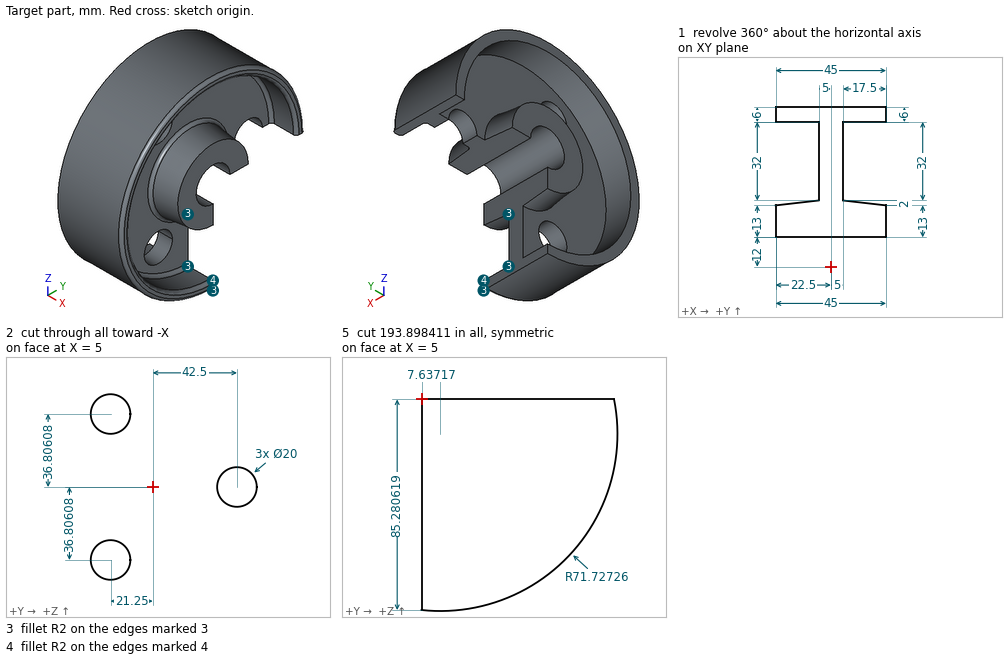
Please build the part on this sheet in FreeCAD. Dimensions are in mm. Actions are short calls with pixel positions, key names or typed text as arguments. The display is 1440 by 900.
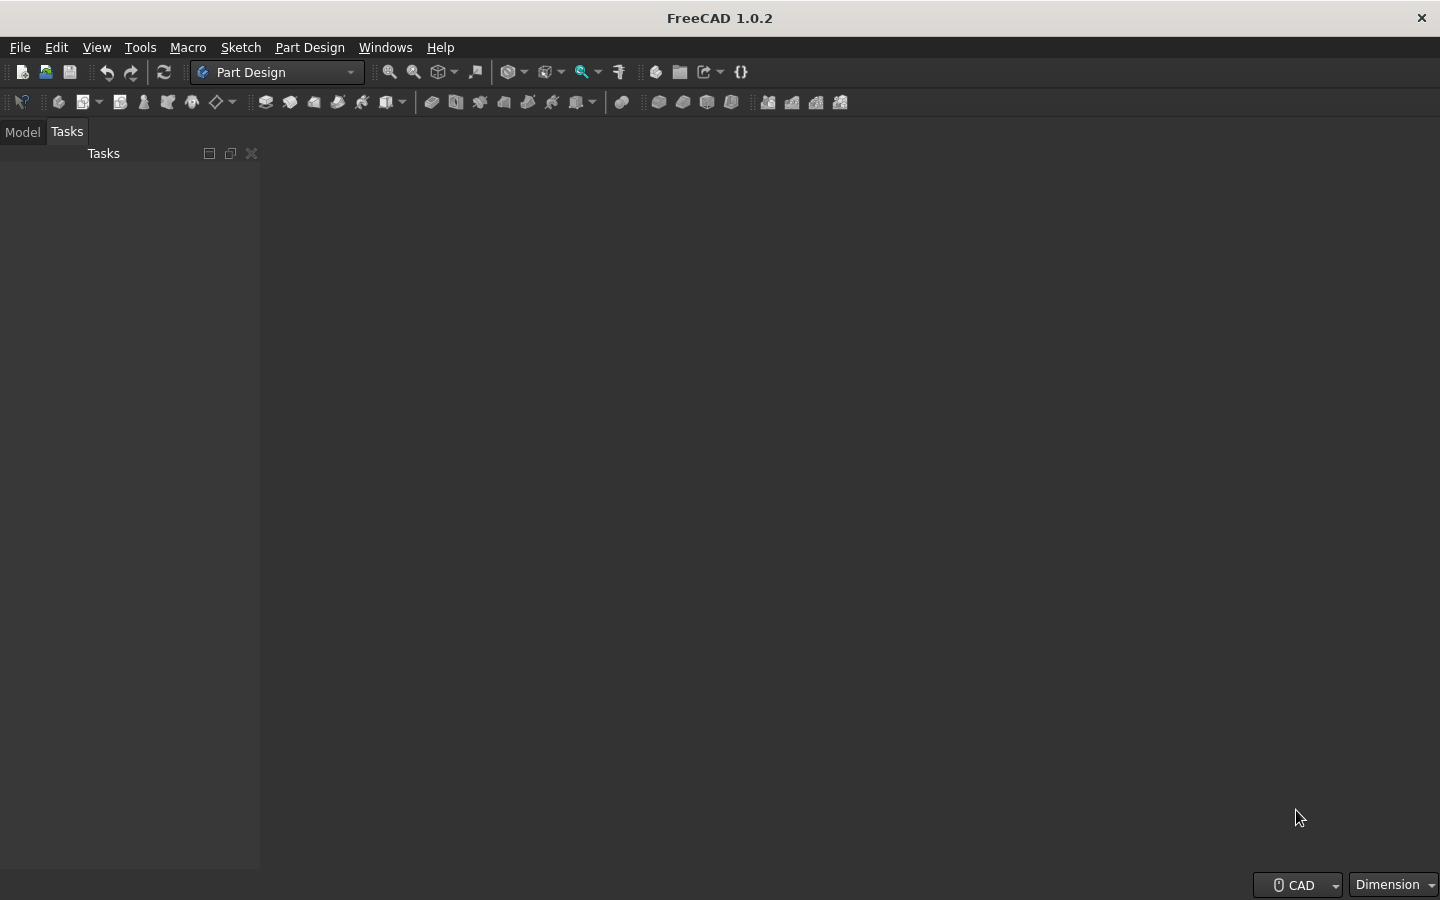
click(22, 72)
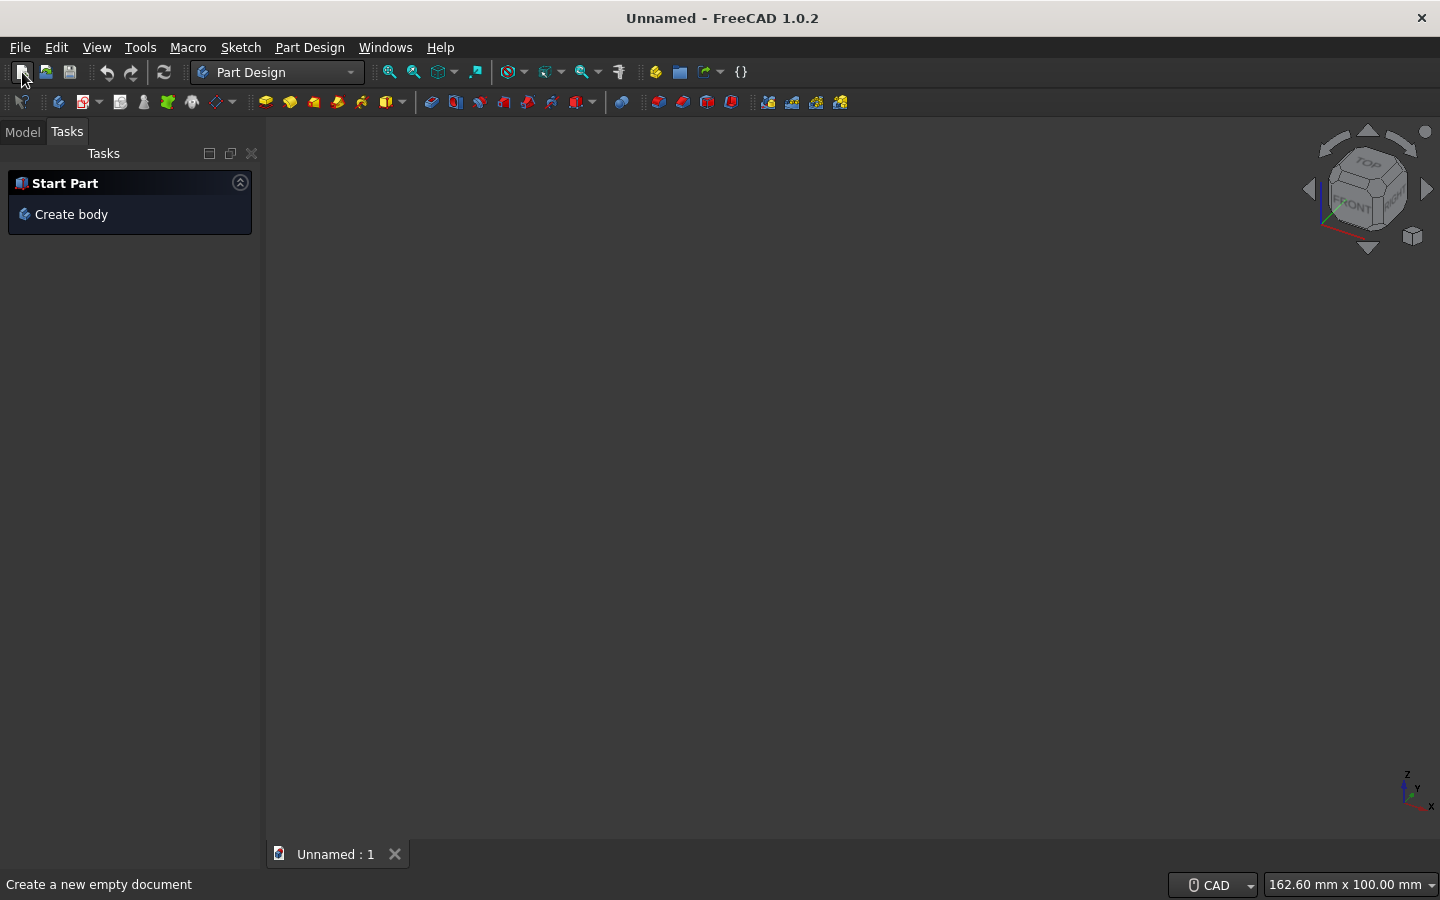
click(84, 102)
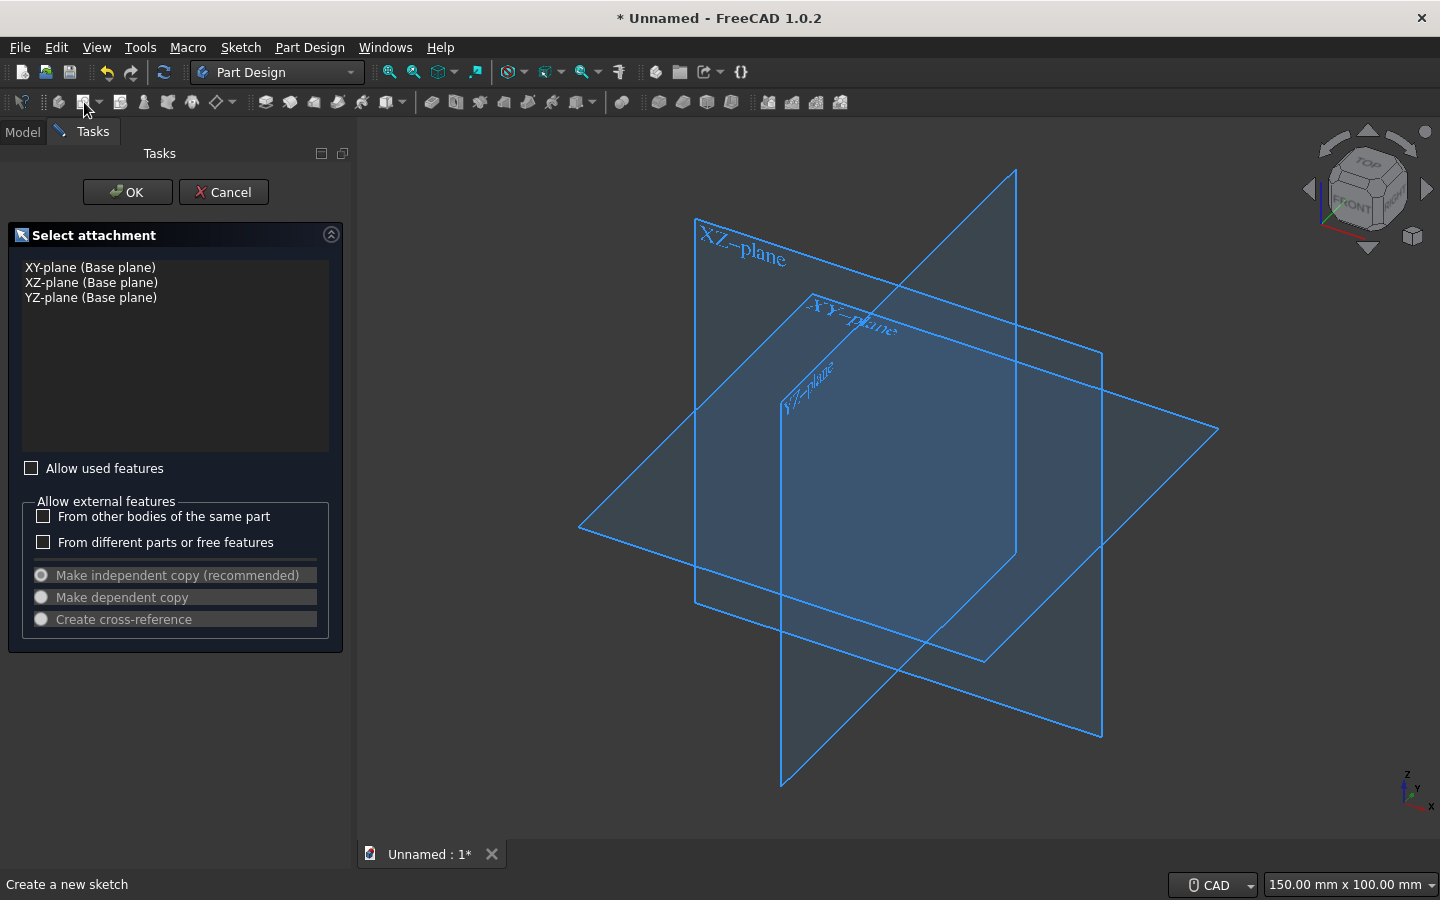
click(82, 268)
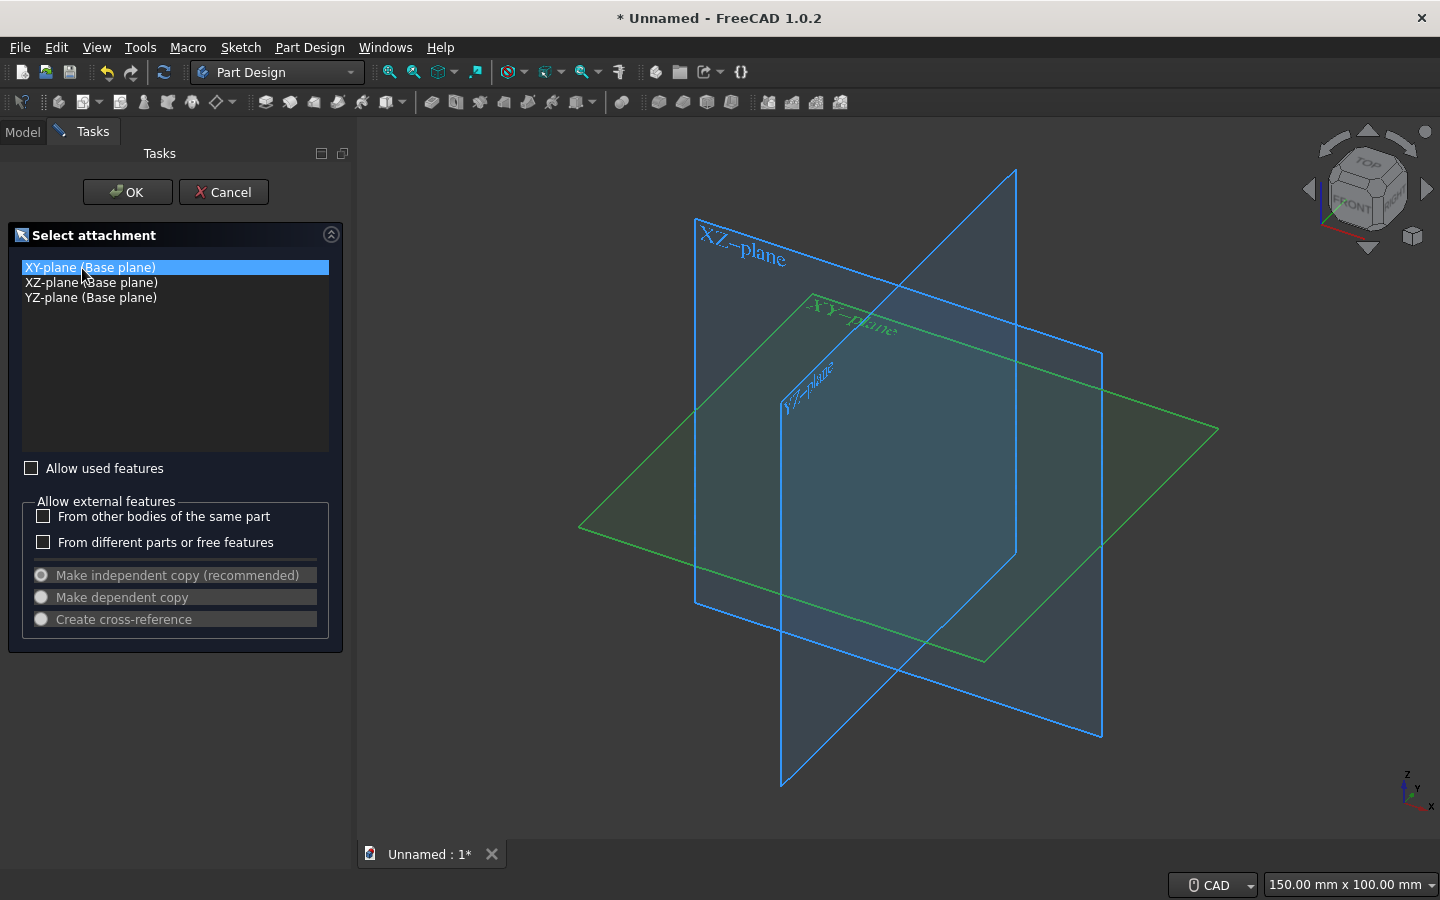
click(128, 192)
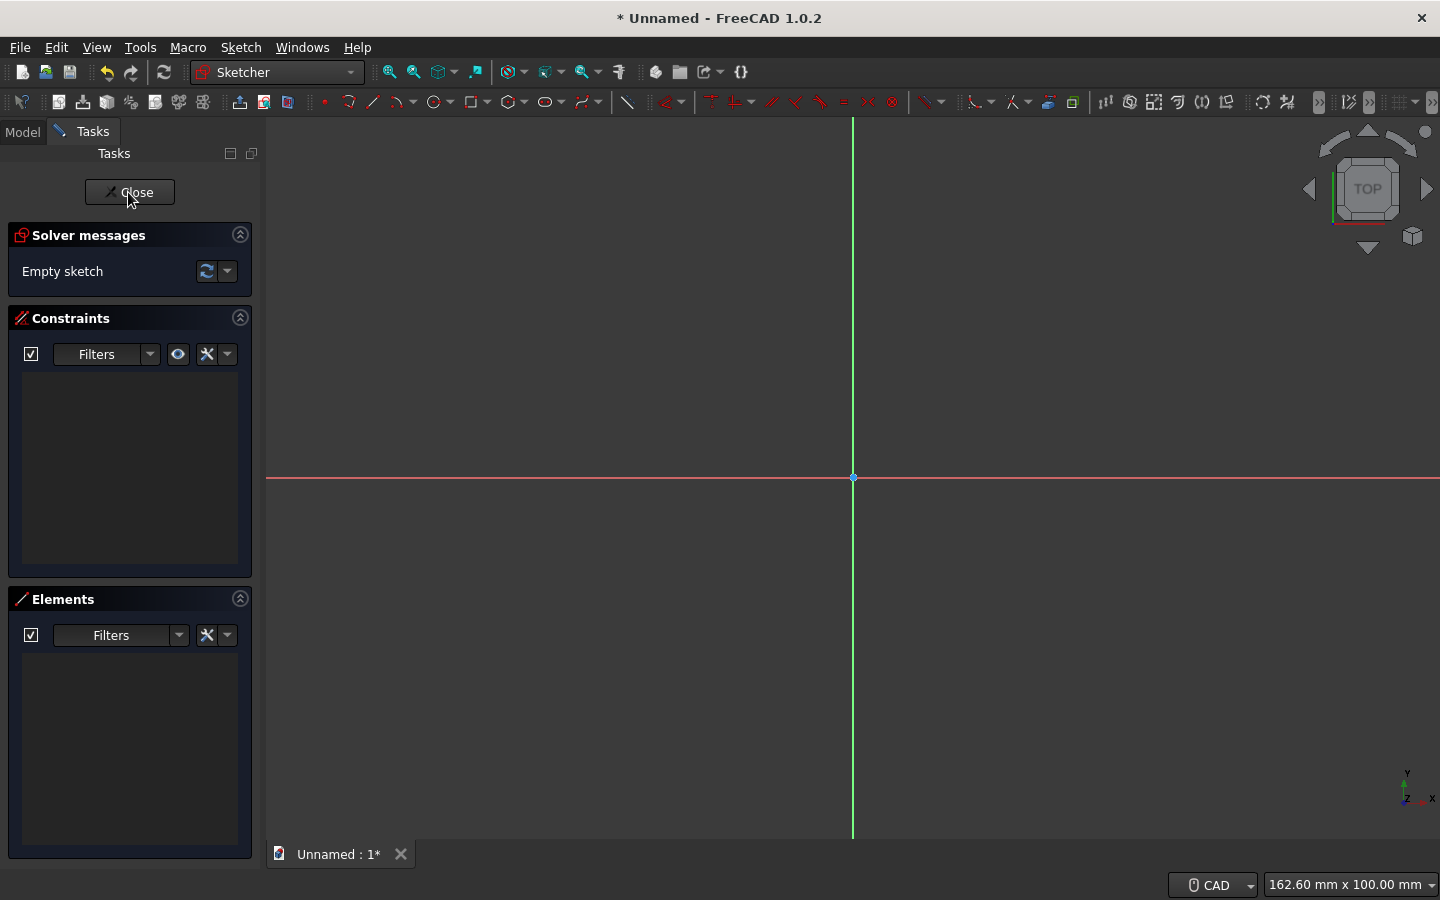
scroll(645, 811, down, 2)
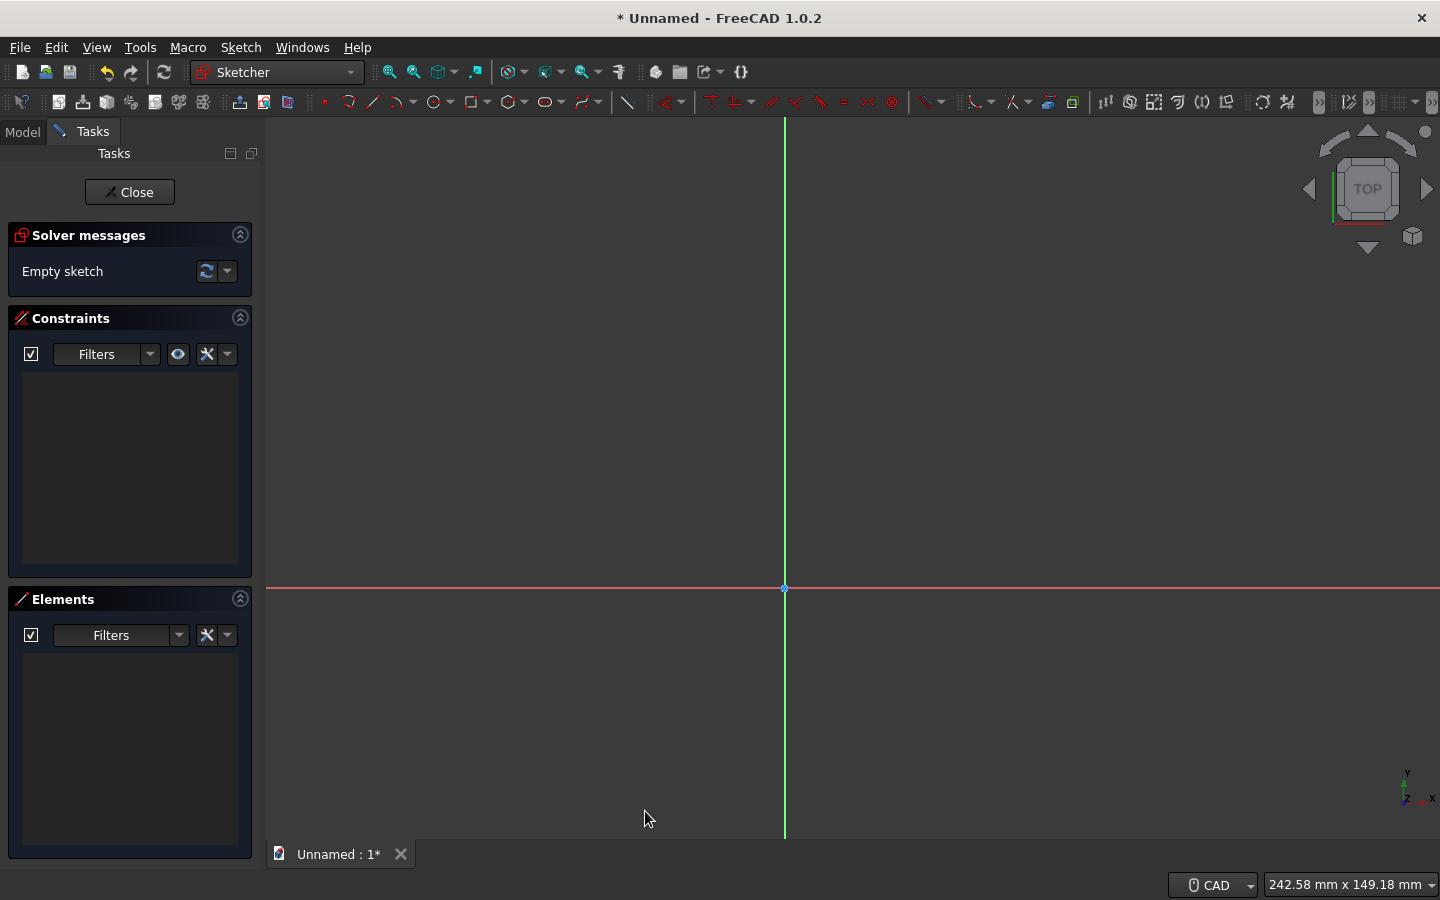
scroll(785, 335, up, 2)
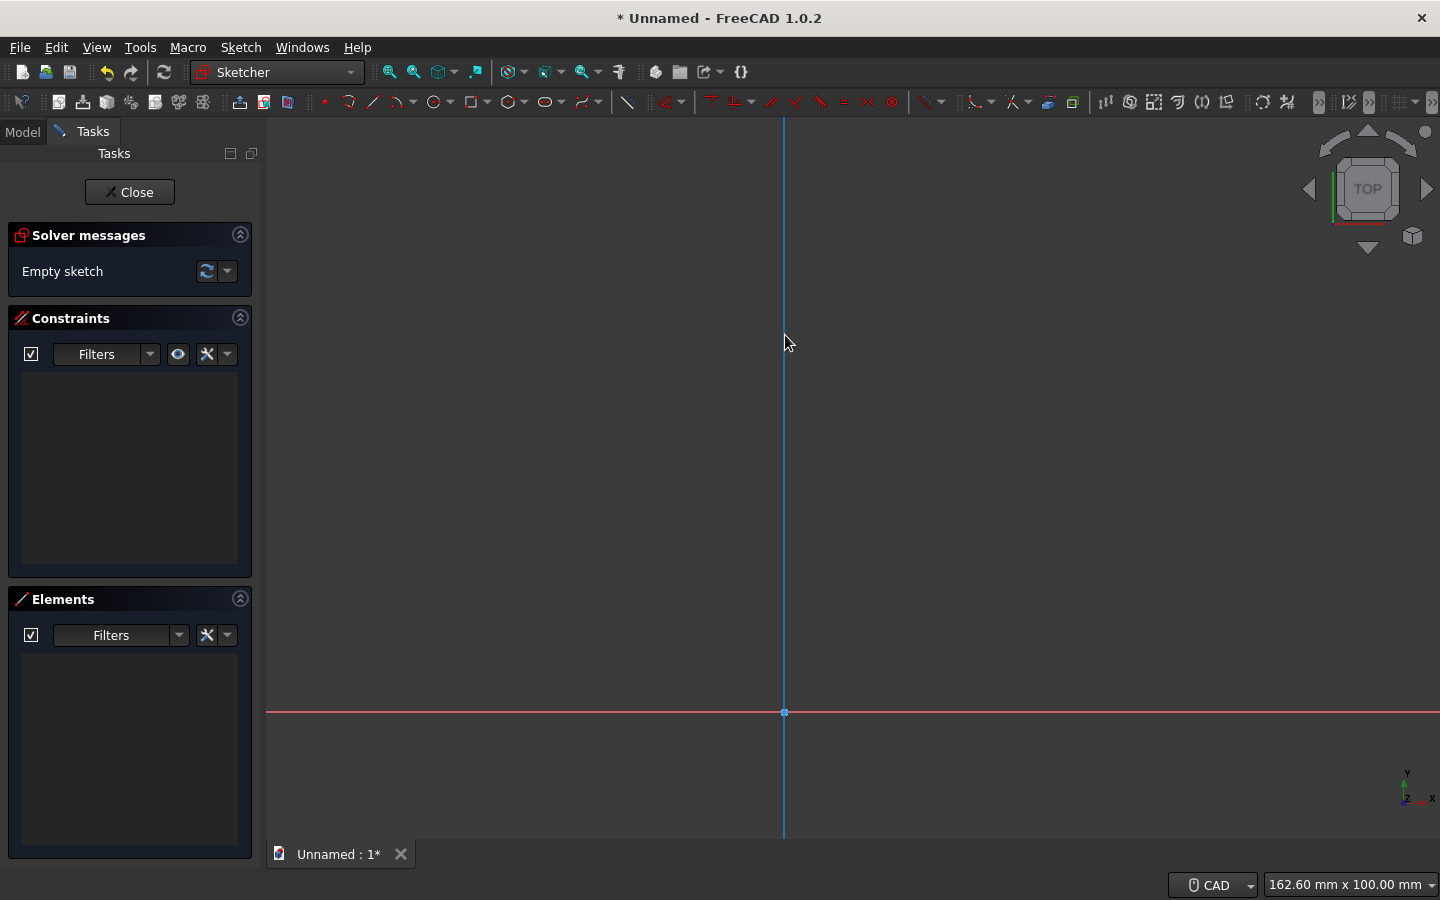
click(350, 102)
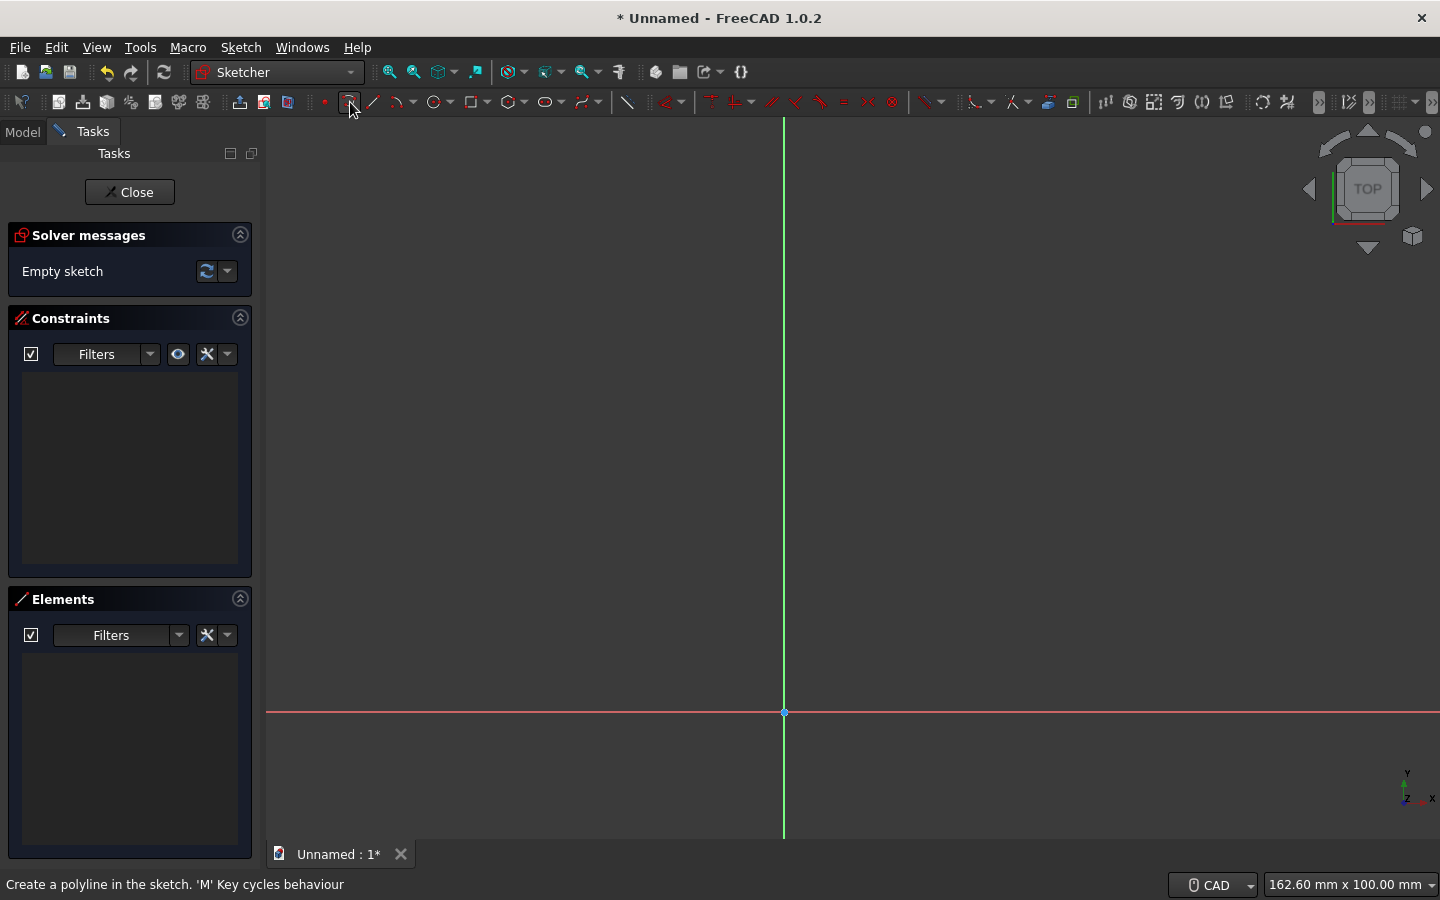
click(622, 626)
click(947, 626)
click(947, 532)
click(820, 517)
click(820, 286)
click(947, 286)
click(947, 243)
click(622, 243)
click(622, 286)
click(748, 286)
click(748, 517)
click(622, 532)
click(622, 627)
key(Escape)
key(Escape)